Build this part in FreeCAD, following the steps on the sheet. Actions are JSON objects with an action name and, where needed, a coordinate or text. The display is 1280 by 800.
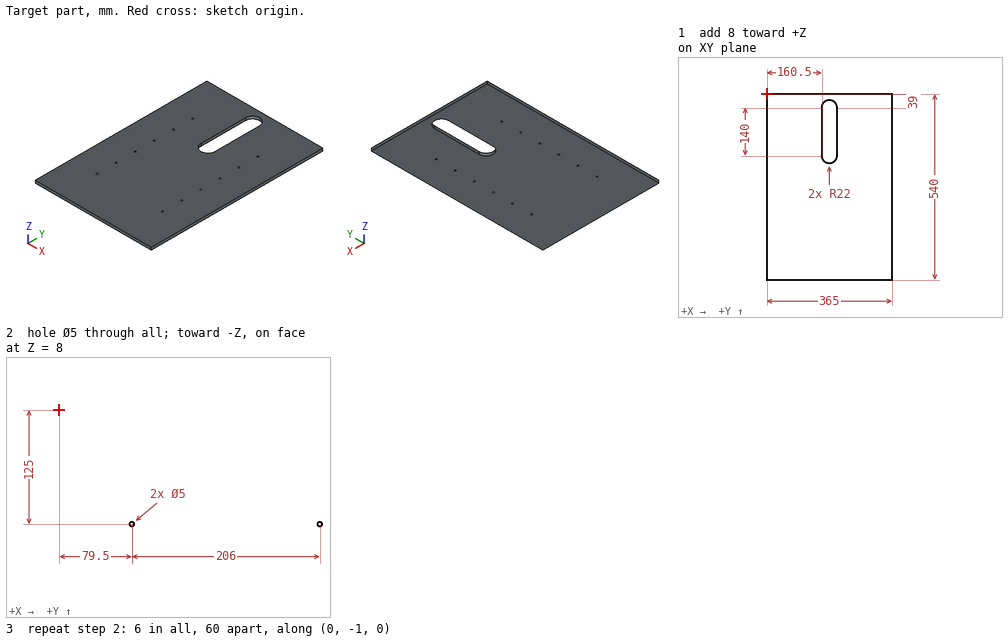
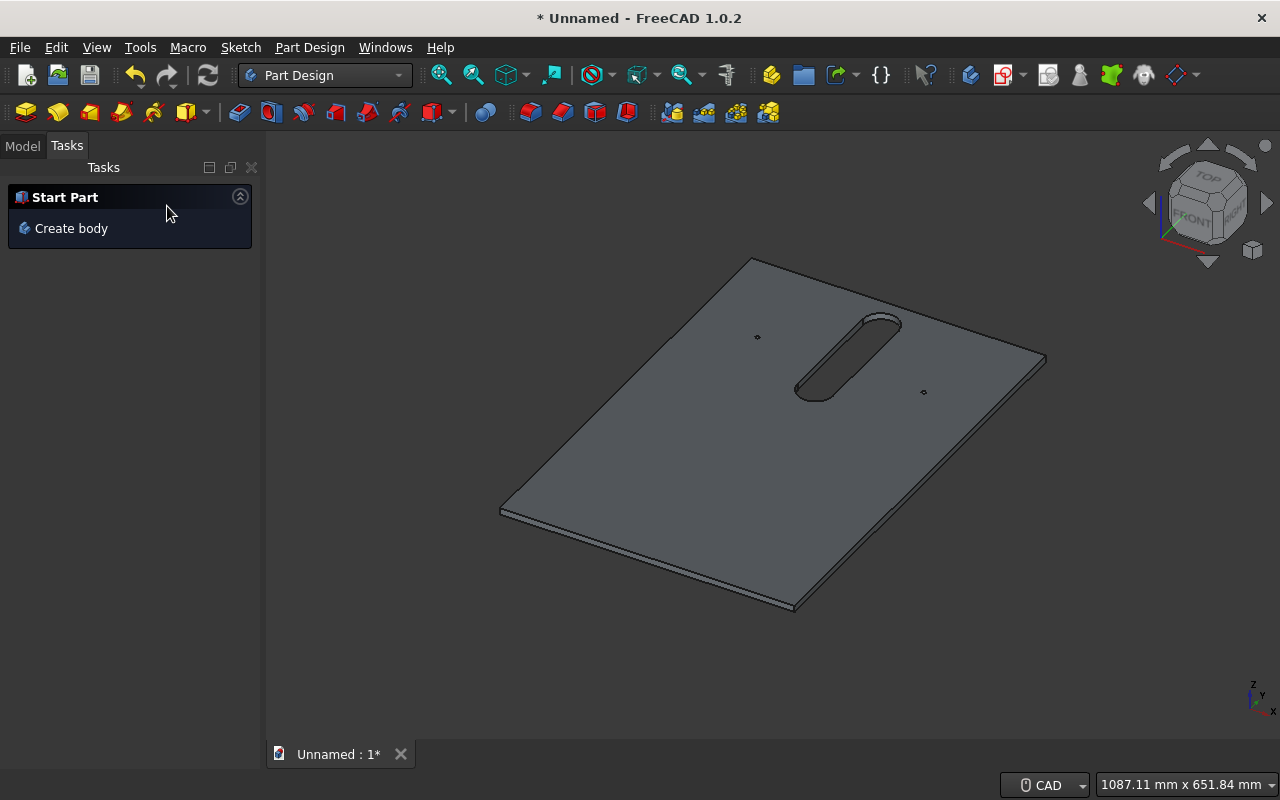
{"action": "left_click", "coordinate": [23, 145]}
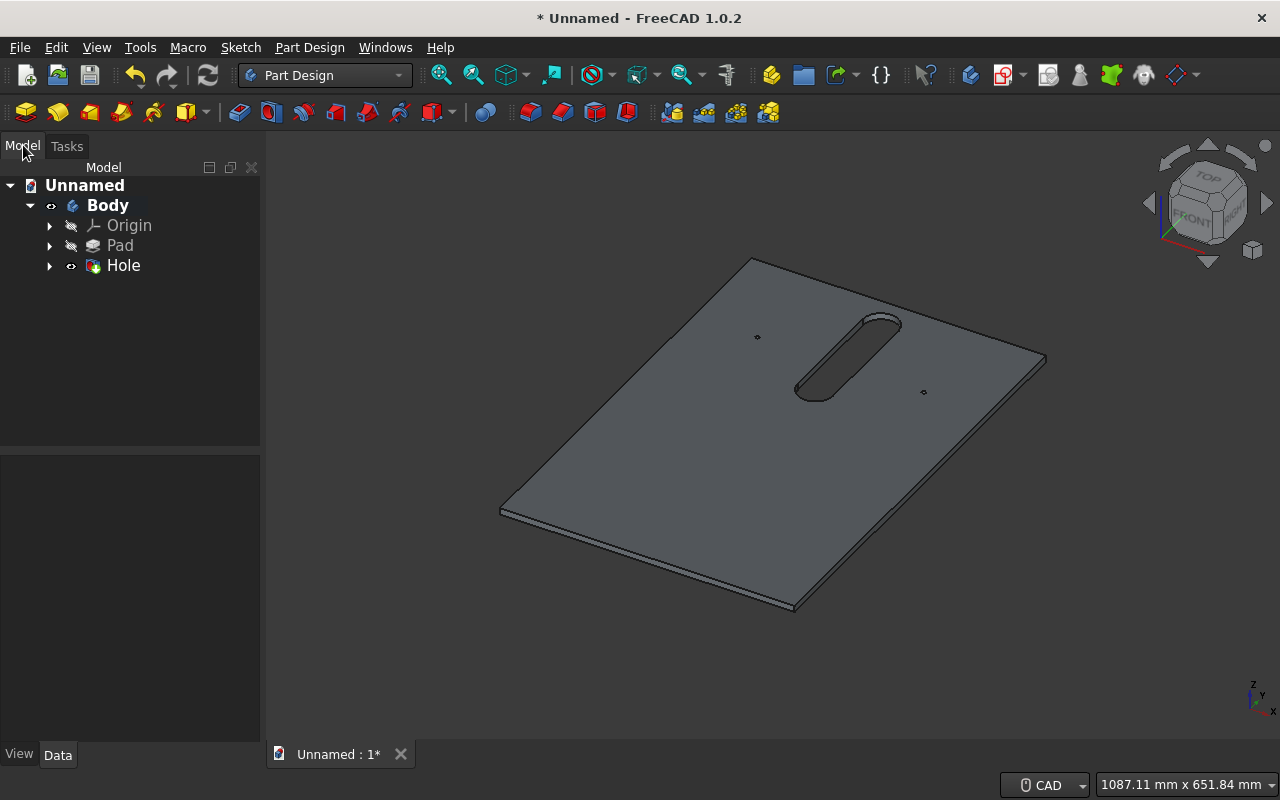
{"action": "left_click", "coordinate": [116, 266]}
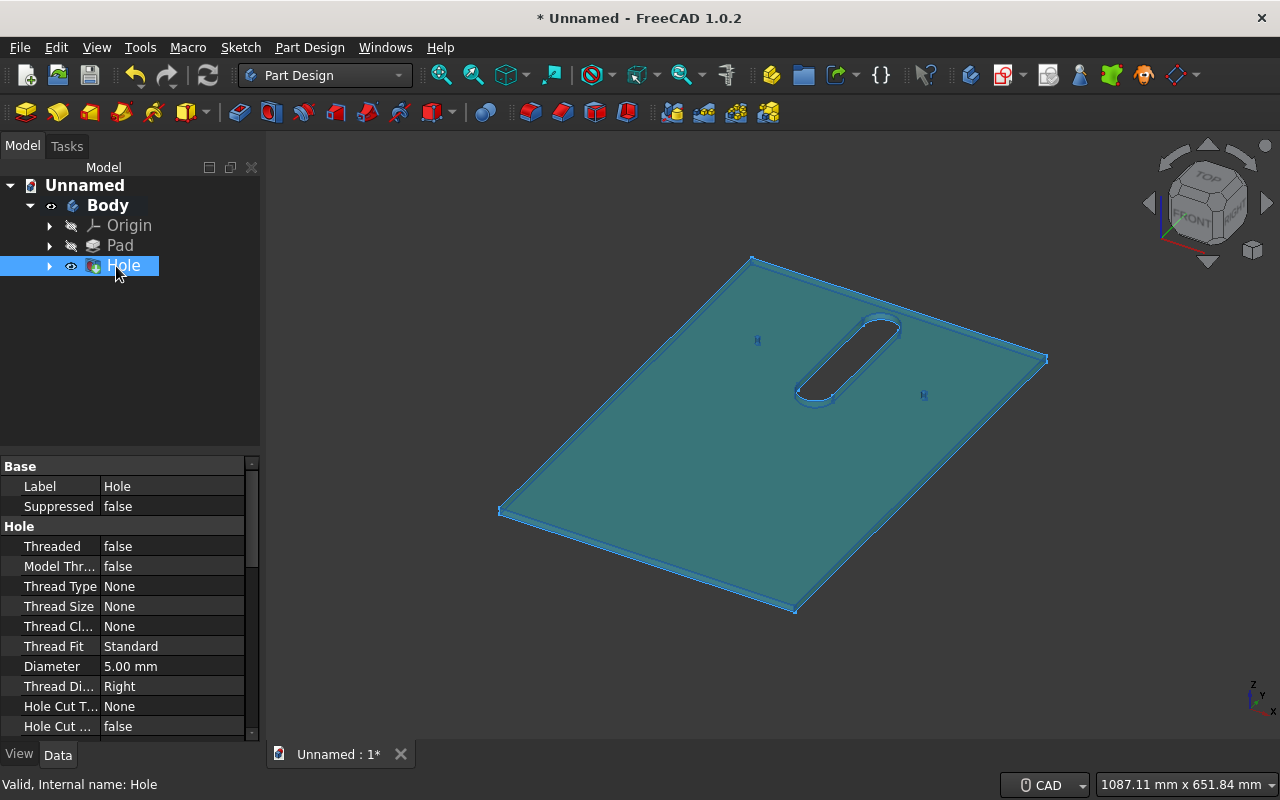
{"action": "left_click", "coordinate": [704, 112]}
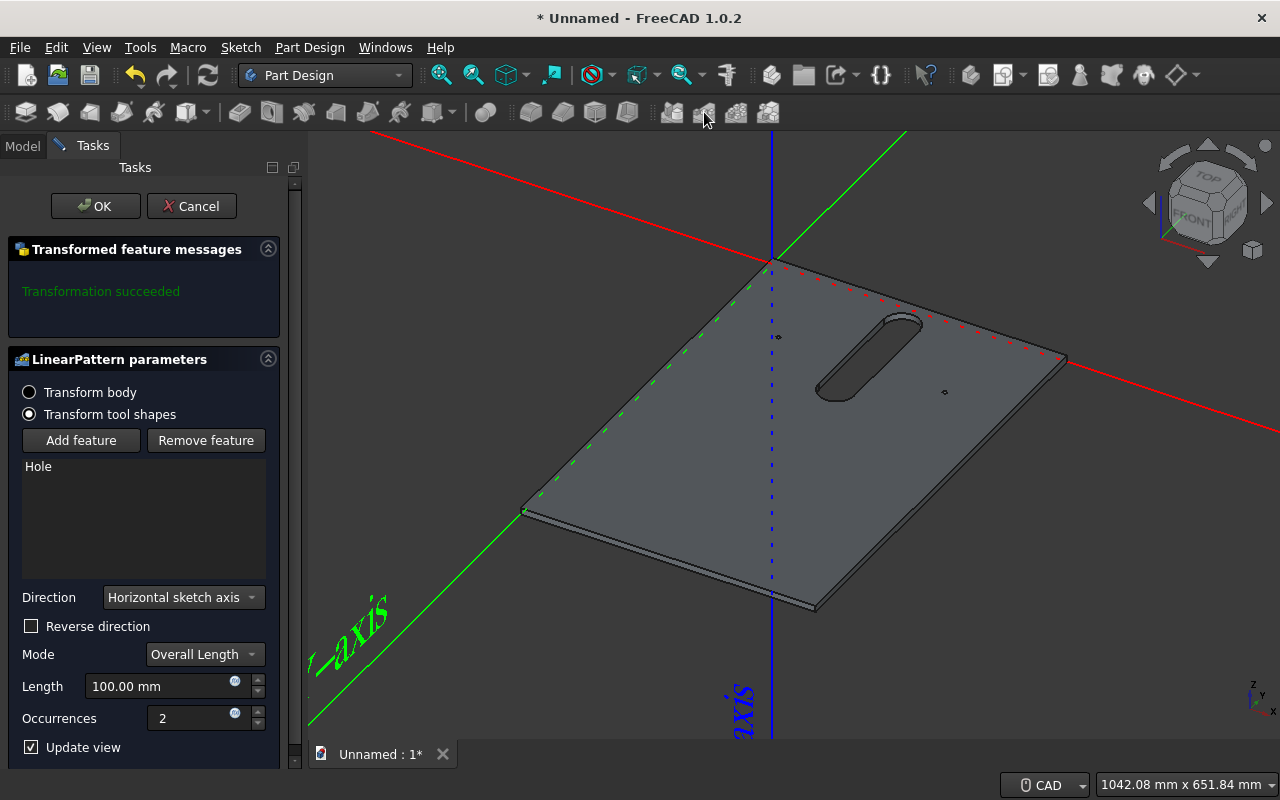
{"action": "left_click", "coordinate": [184, 598]}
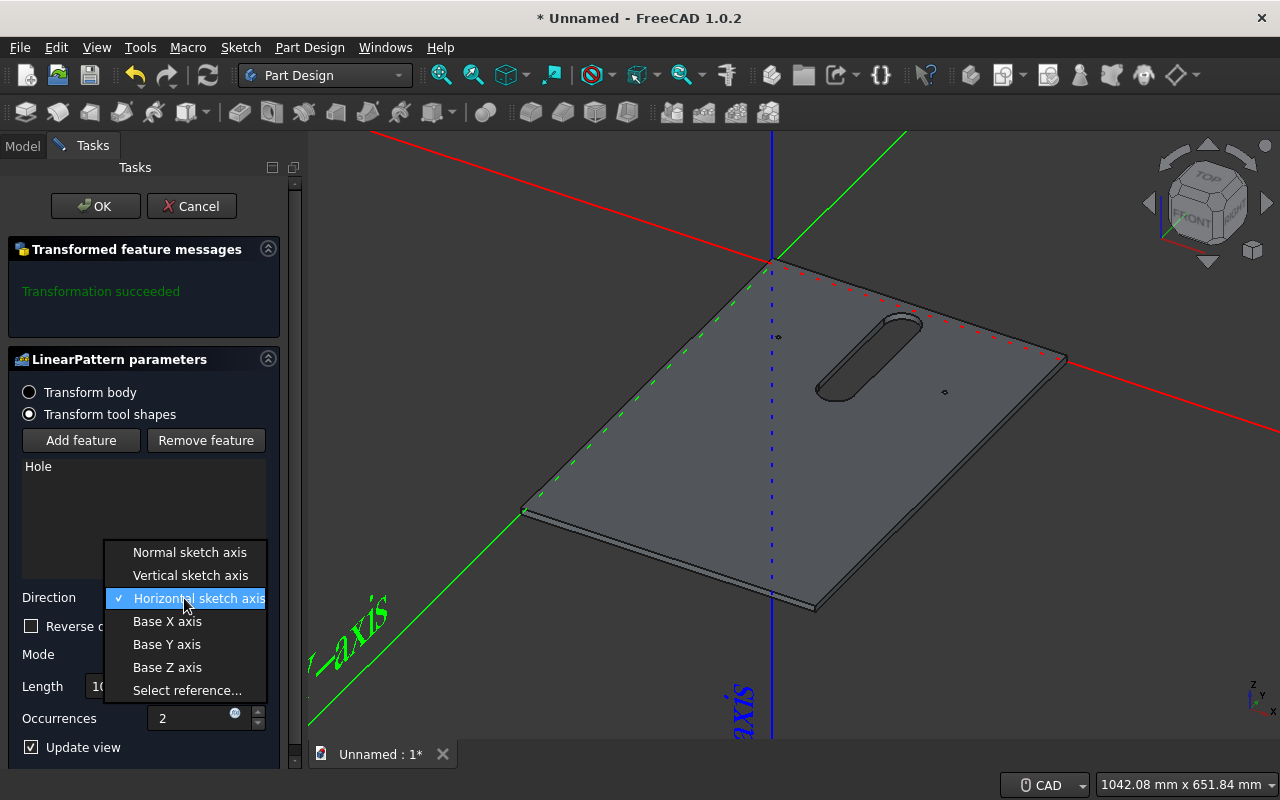
{"action": "left_click", "coordinate": [184, 644]}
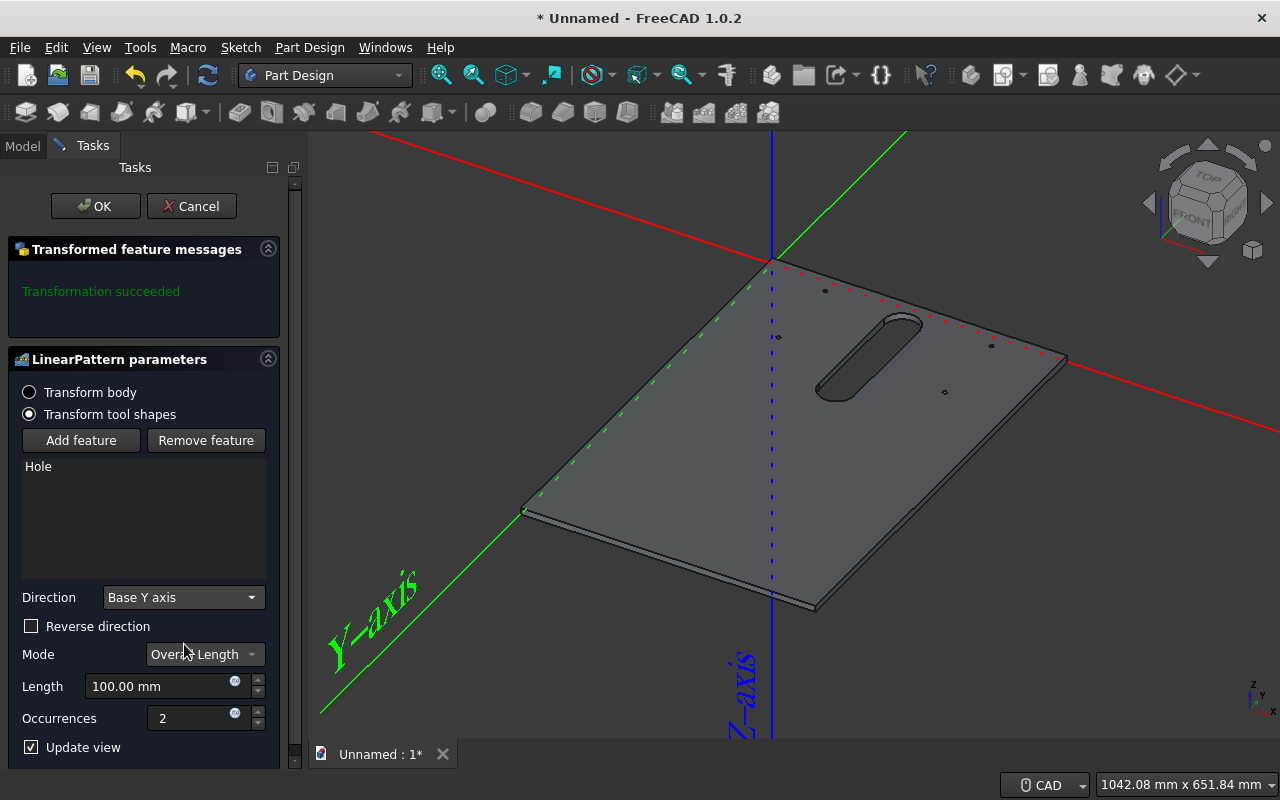
{"action": "left_click", "coordinate": [206, 654]}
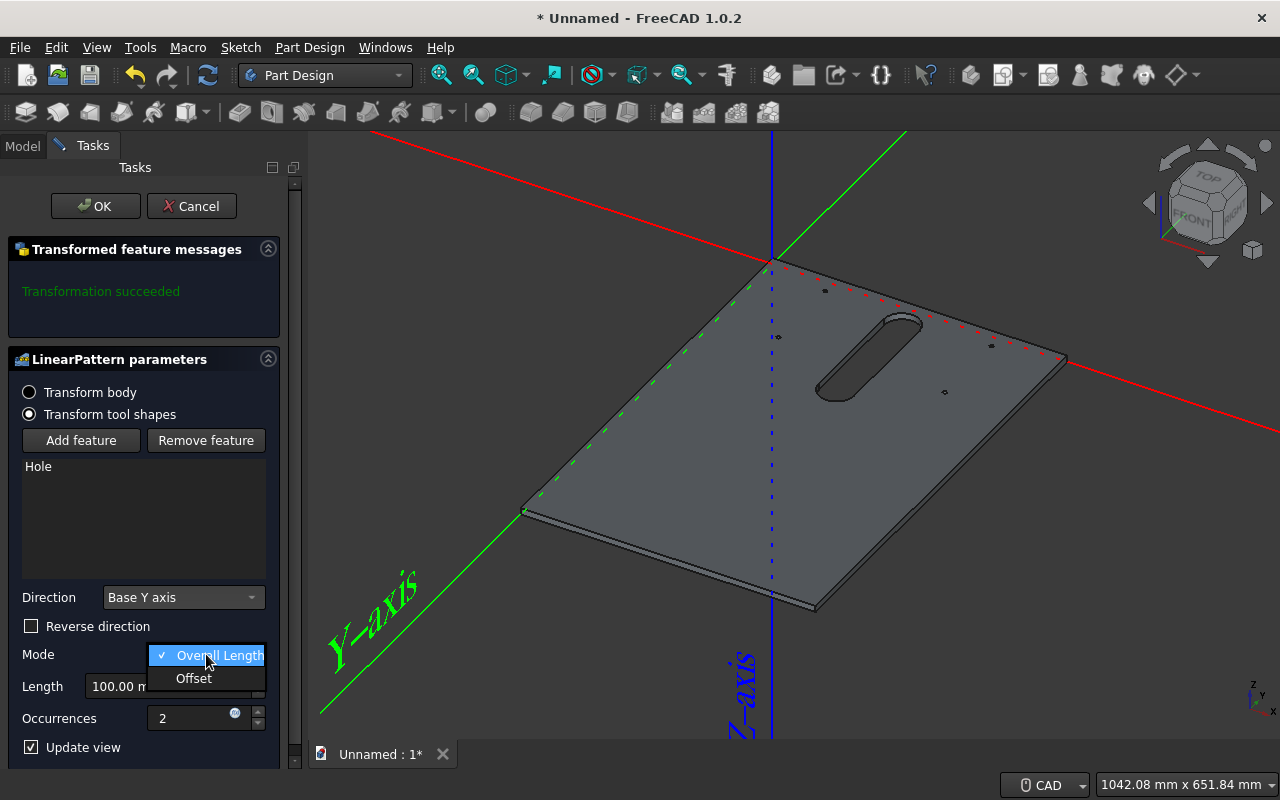
{"action": "left_click", "coordinate": [206, 678]}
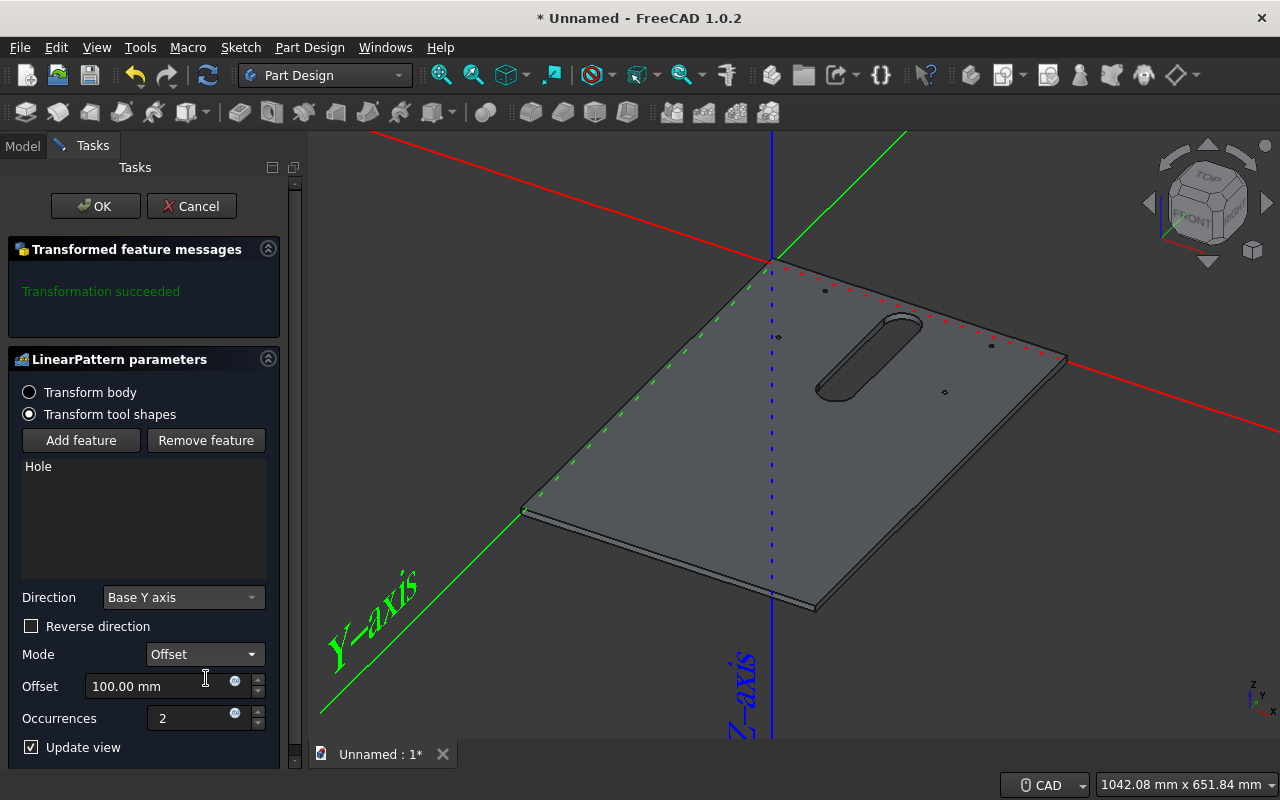
{"action": "triple_click", "coordinate": [168, 686]}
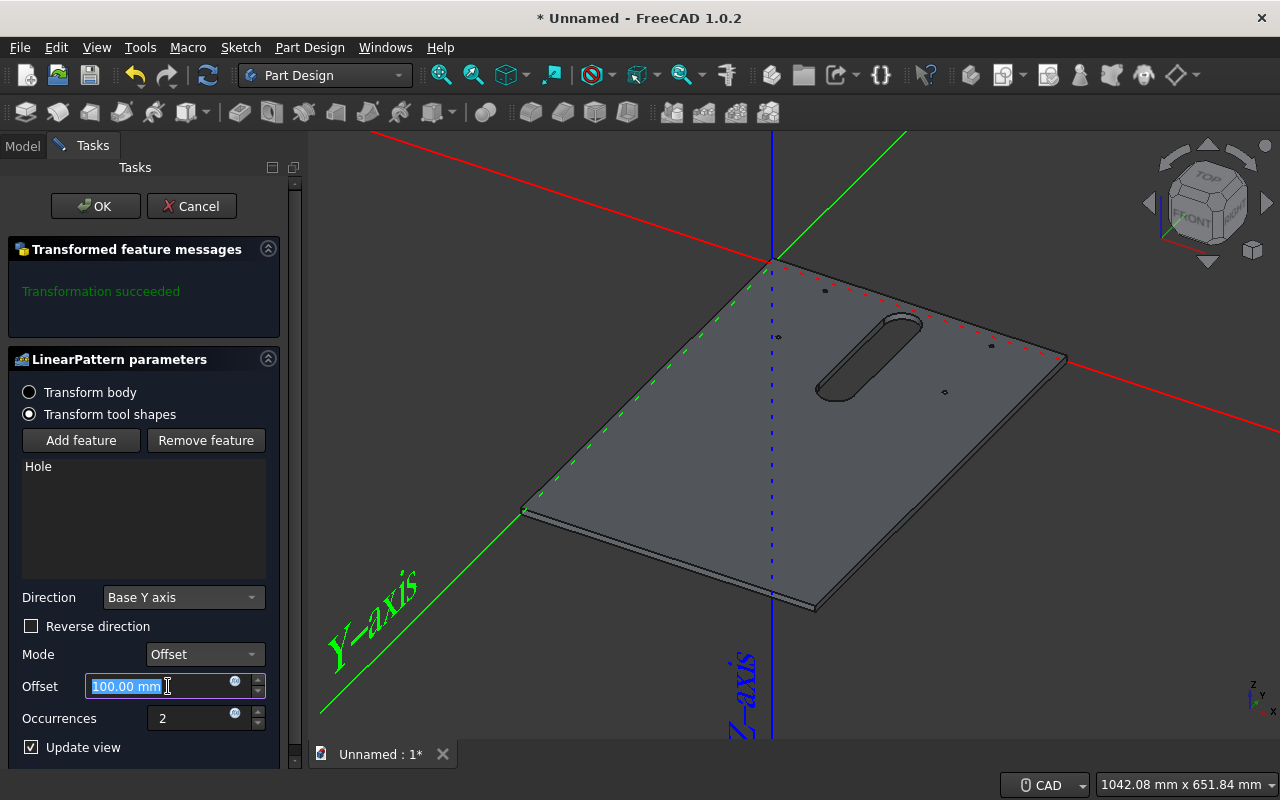
{"action": "type", "text": "60"}
{"action": "key", "text": "Tab"}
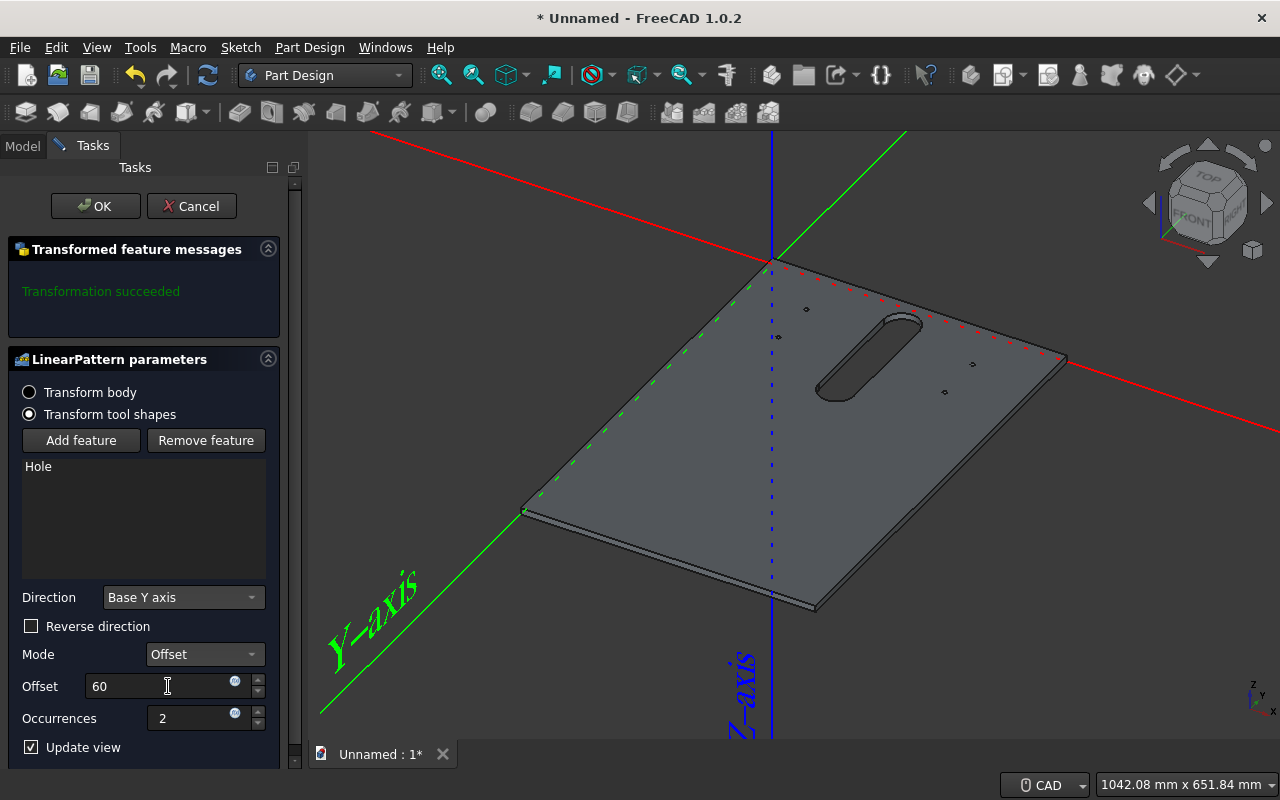
{"action": "triple_click", "coordinate": [198, 718]}